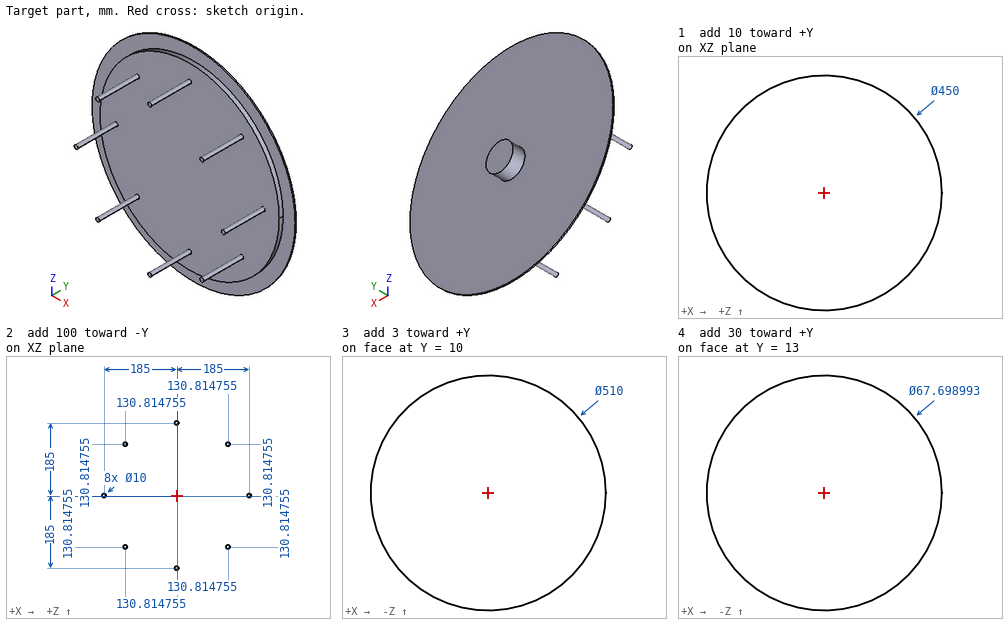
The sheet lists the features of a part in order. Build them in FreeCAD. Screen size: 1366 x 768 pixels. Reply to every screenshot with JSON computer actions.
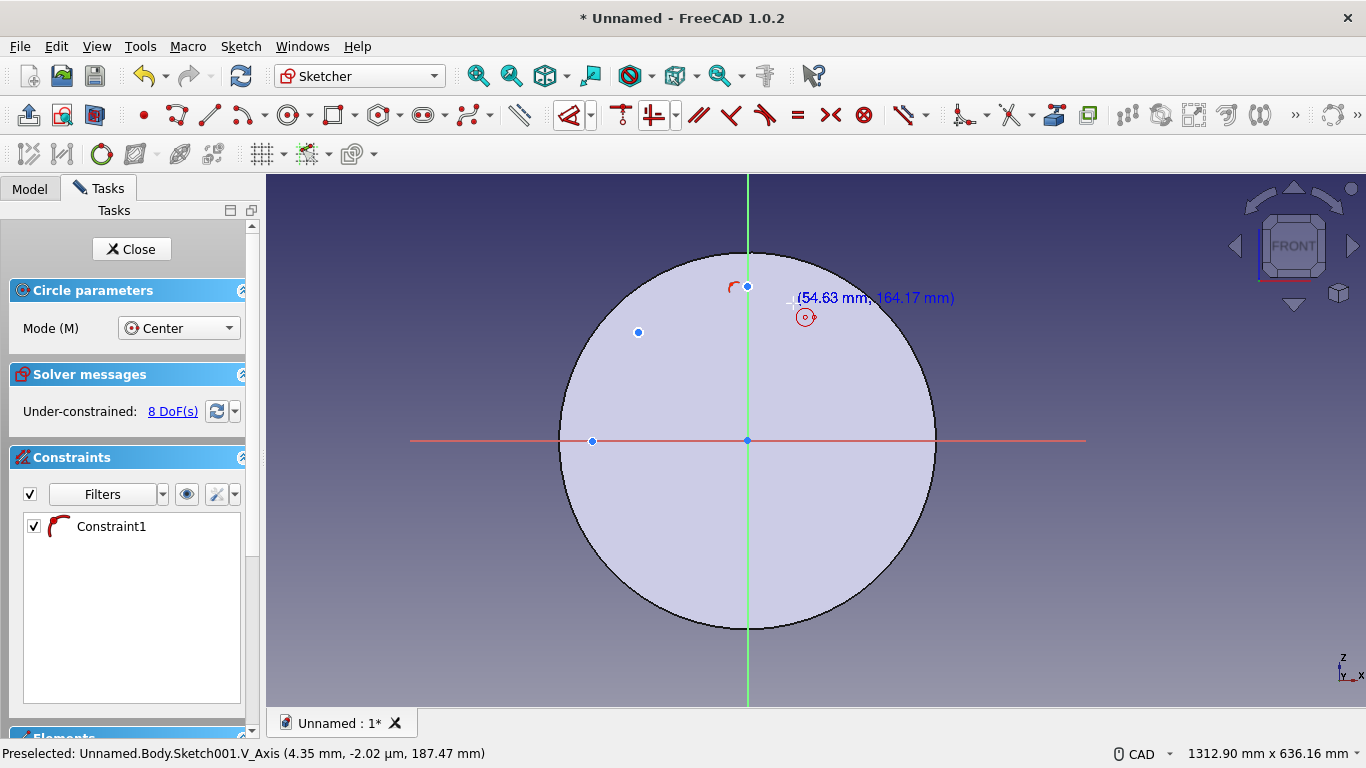
{"action": "left_click", "coordinate": [857, 331]}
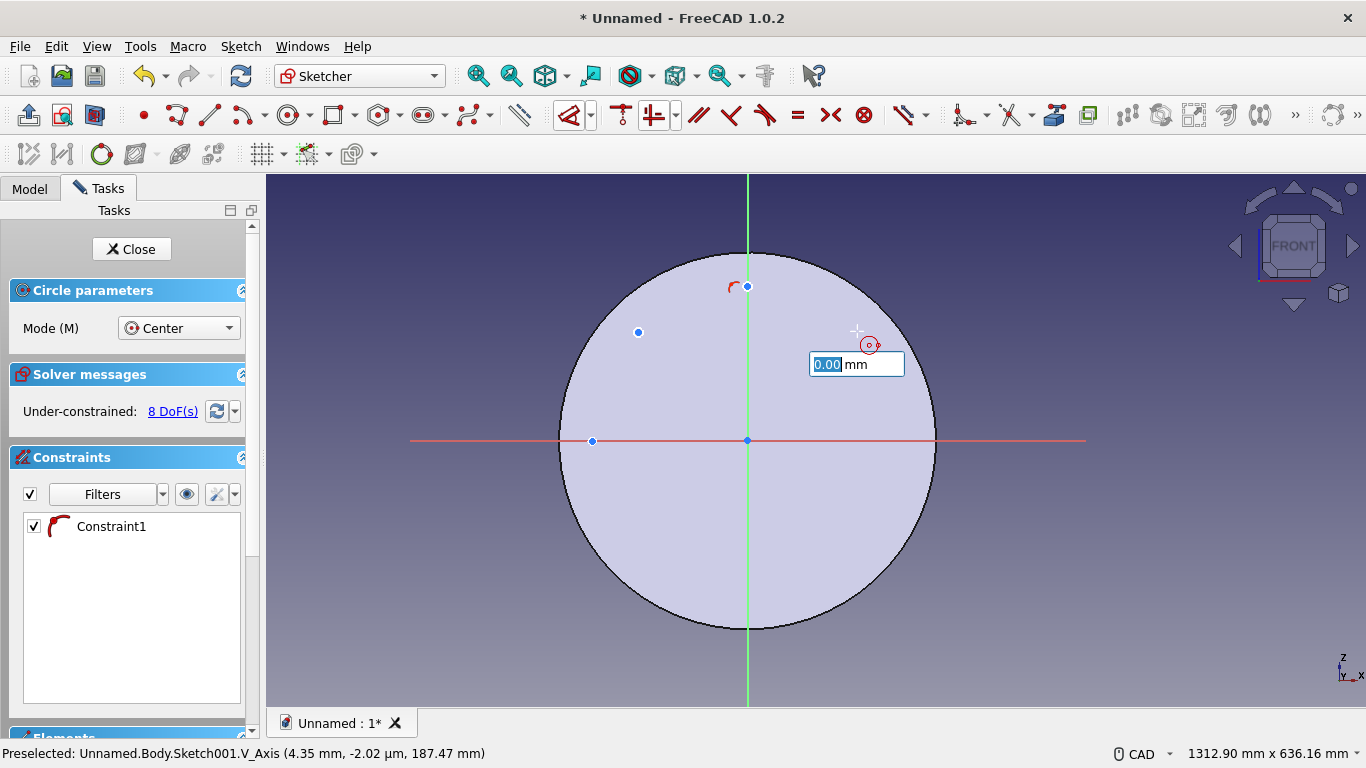
{"action": "scroll", "coordinate": [860, 328], "scroll_direction": "up", "scroll_amount": 7}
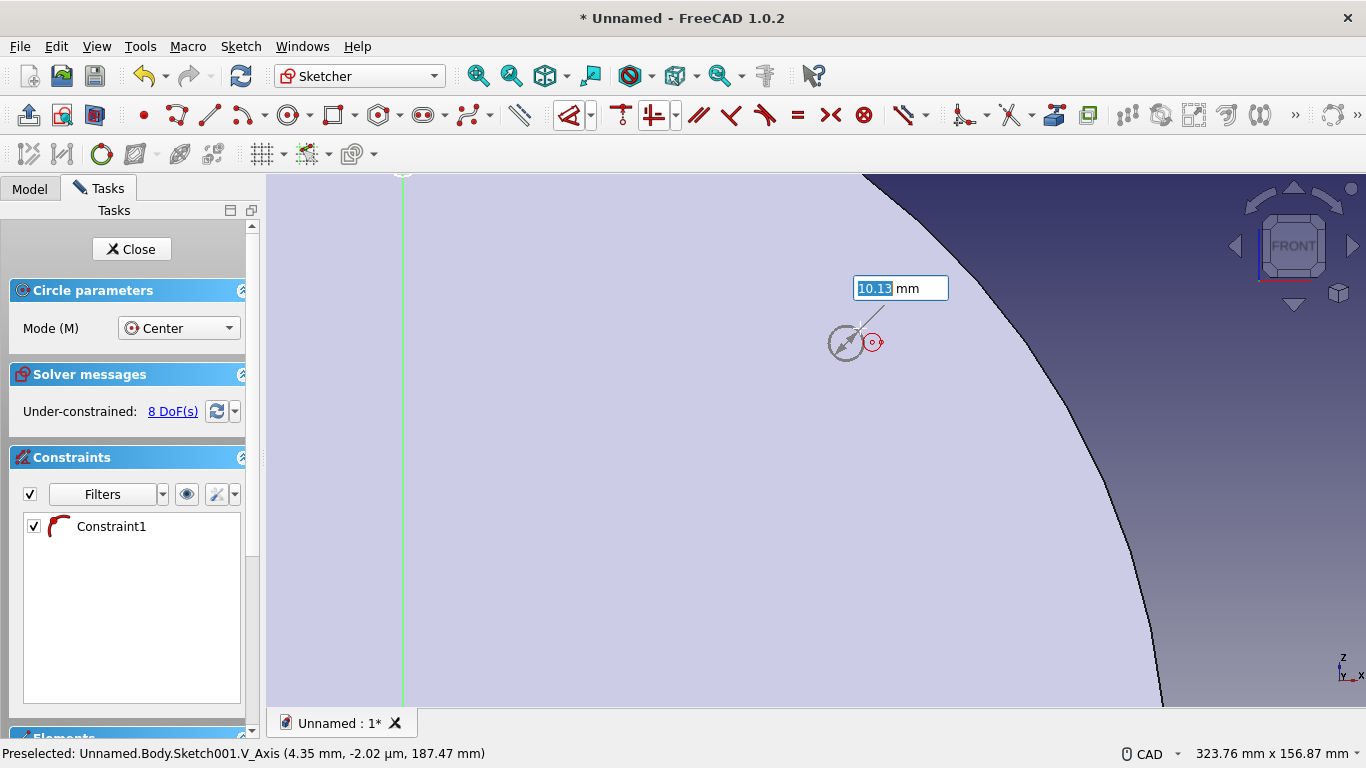
{"action": "left_click", "coordinate": [859, 329]}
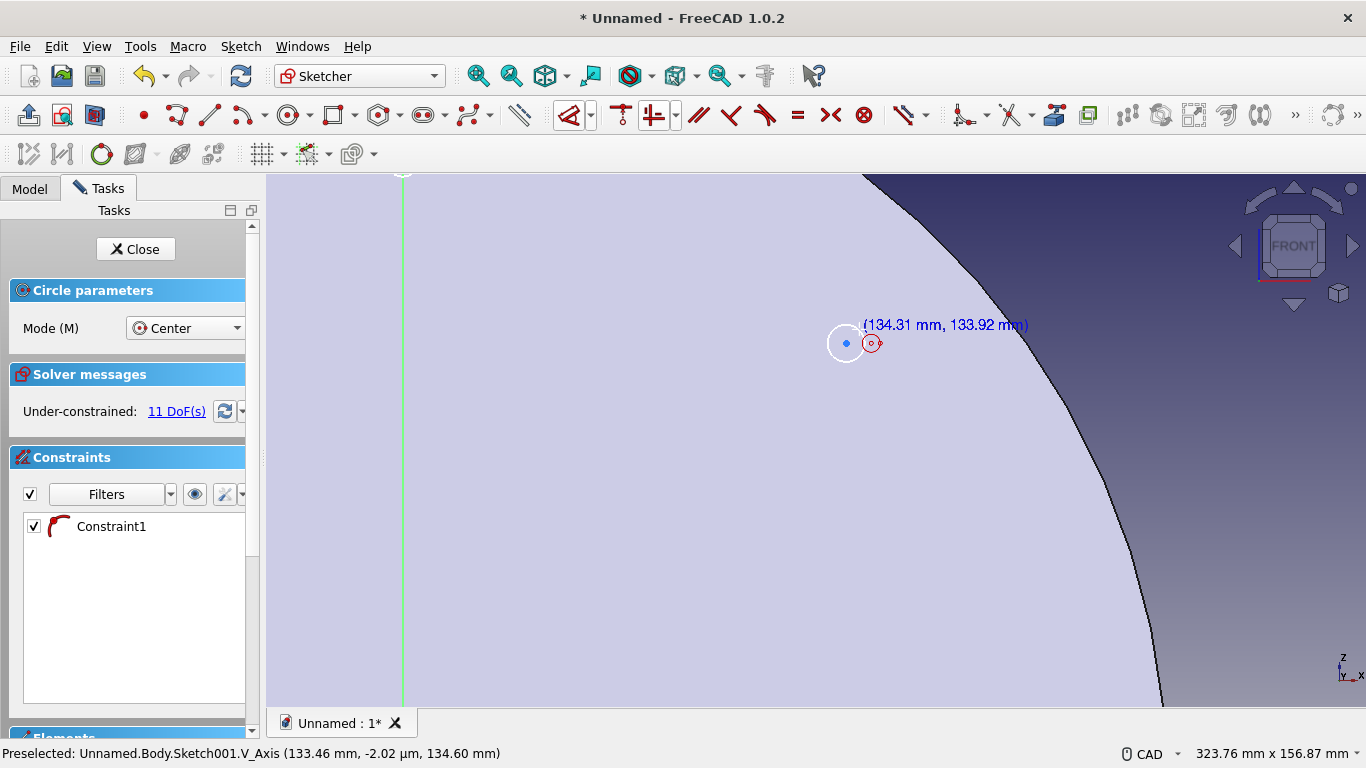
{"action": "scroll", "coordinate": [860, 328], "scroll_direction": "down", "scroll_amount": 7}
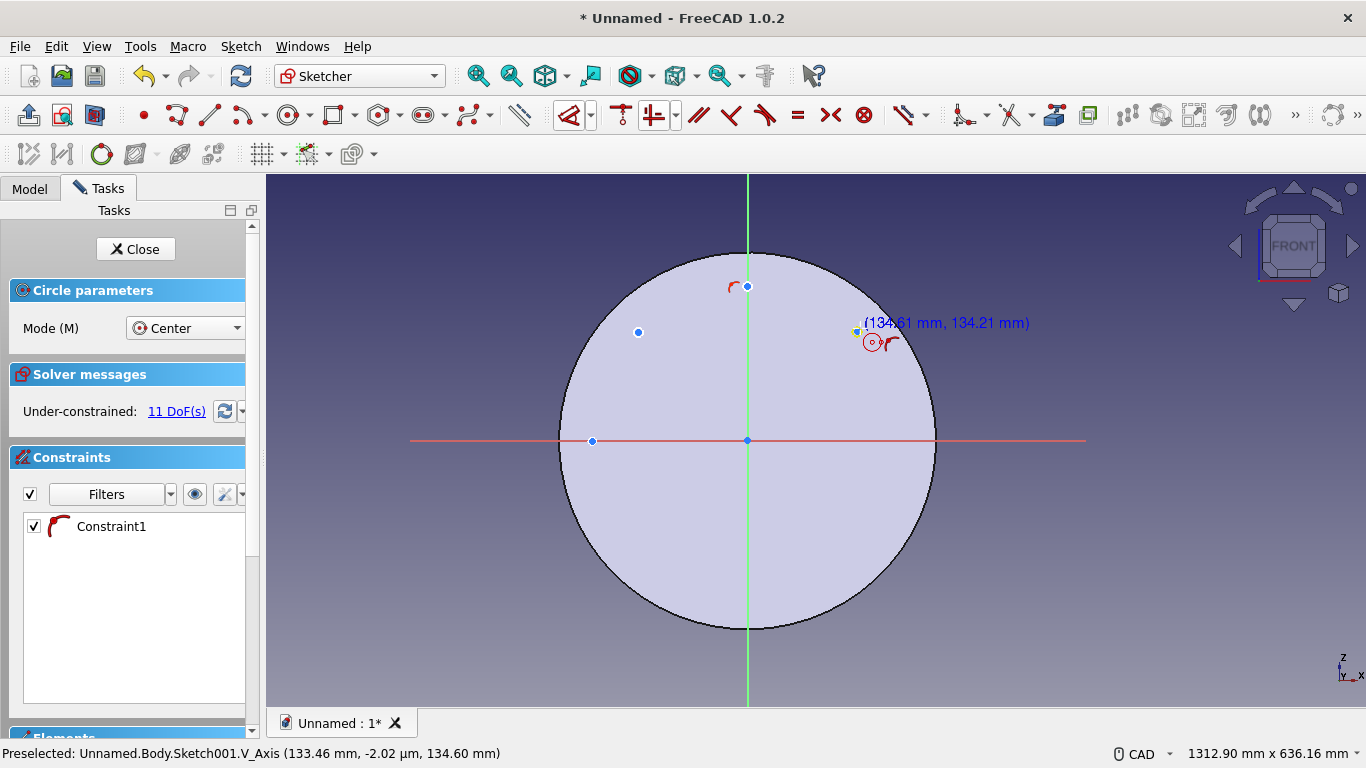
{"action": "scroll", "coordinate": [903, 441], "scroll_direction": "up", "scroll_amount": 9}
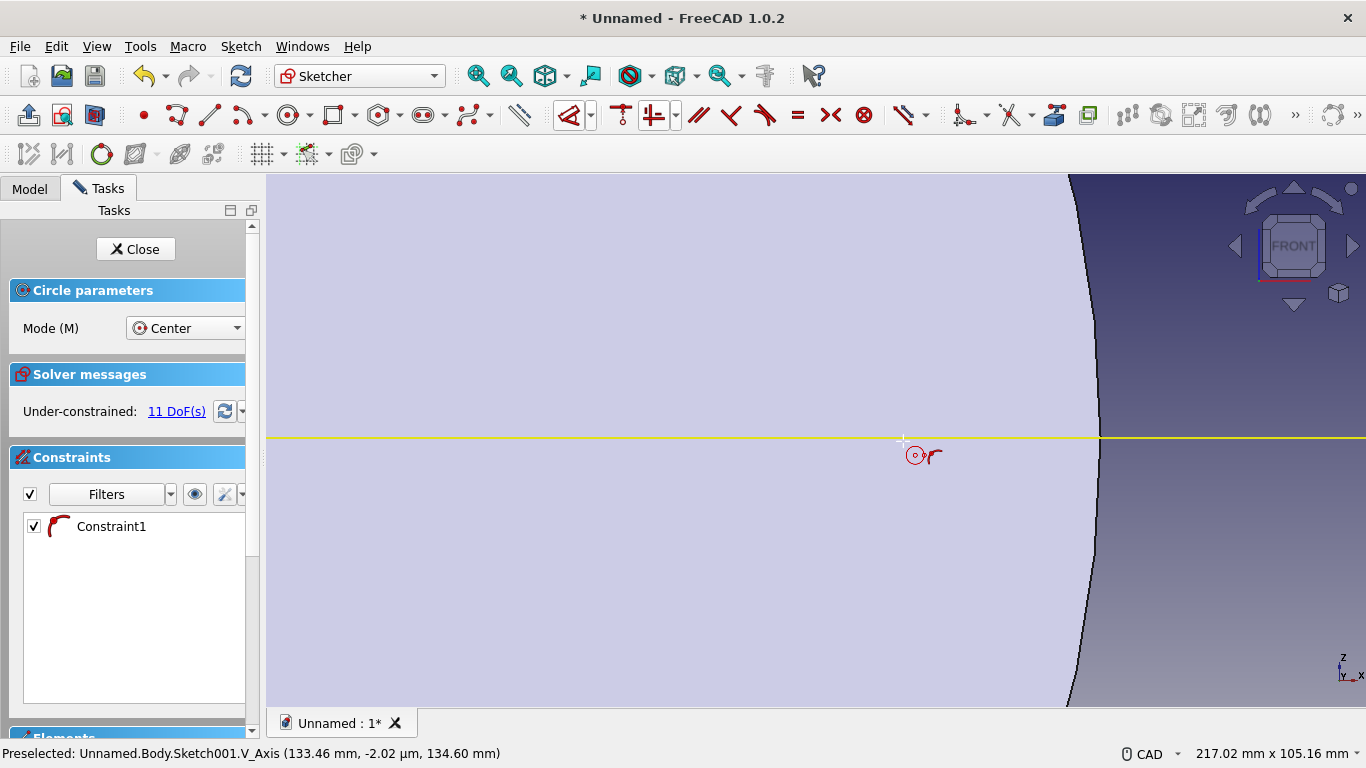
{"action": "scroll", "coordinate": [903, 441], "scroll_direction": "down", "scroll_amount": 9}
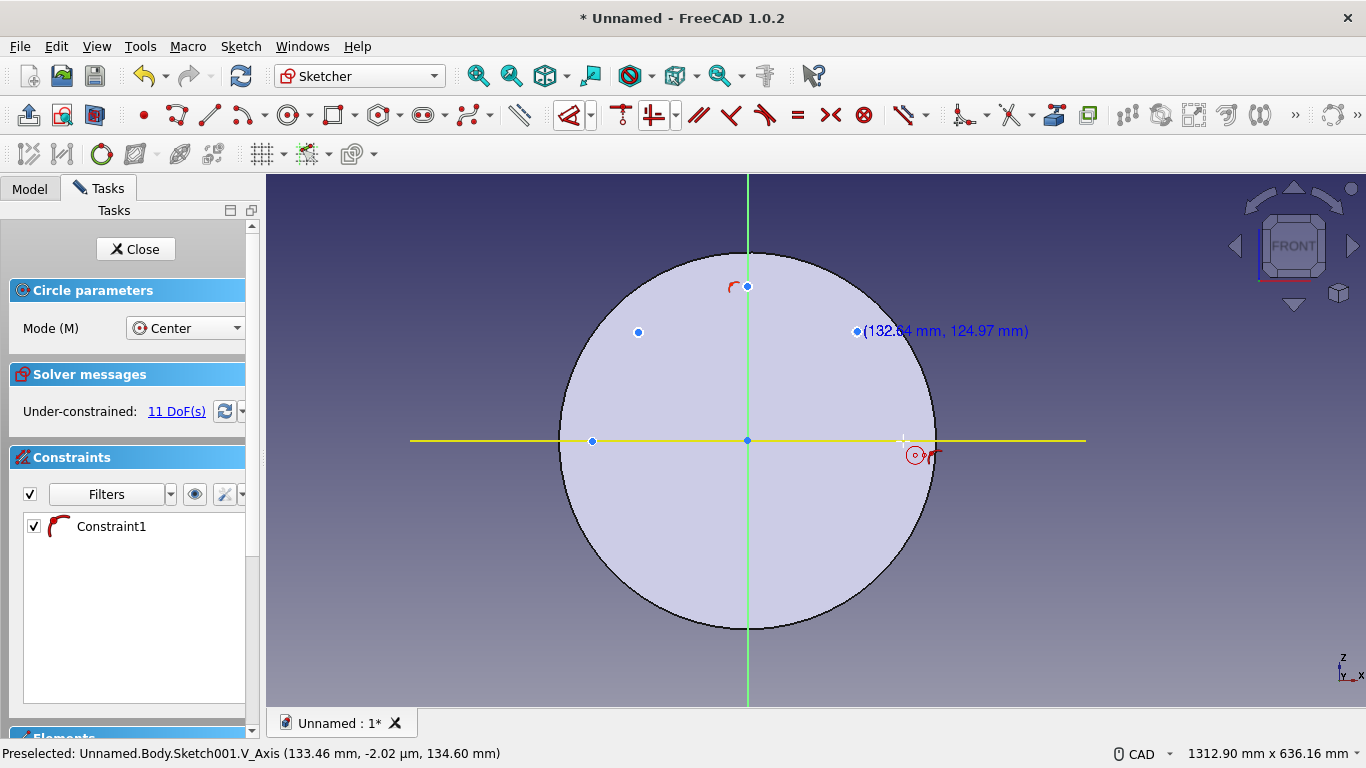
{"action": "left_click", "coordinate": [903, 441]}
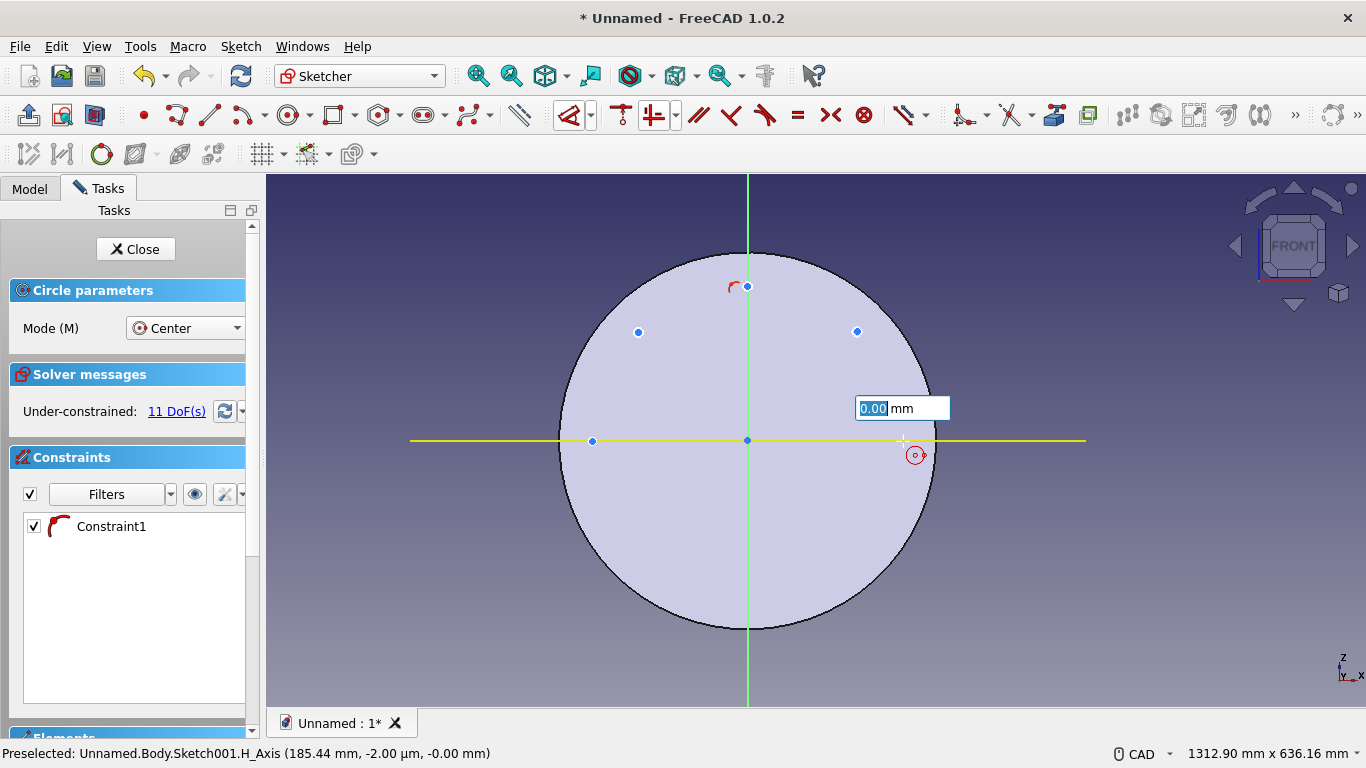
{"action": "scroll", "coordinate": [901, 445], "scroll_direction": "up", "scroll_amount": 7}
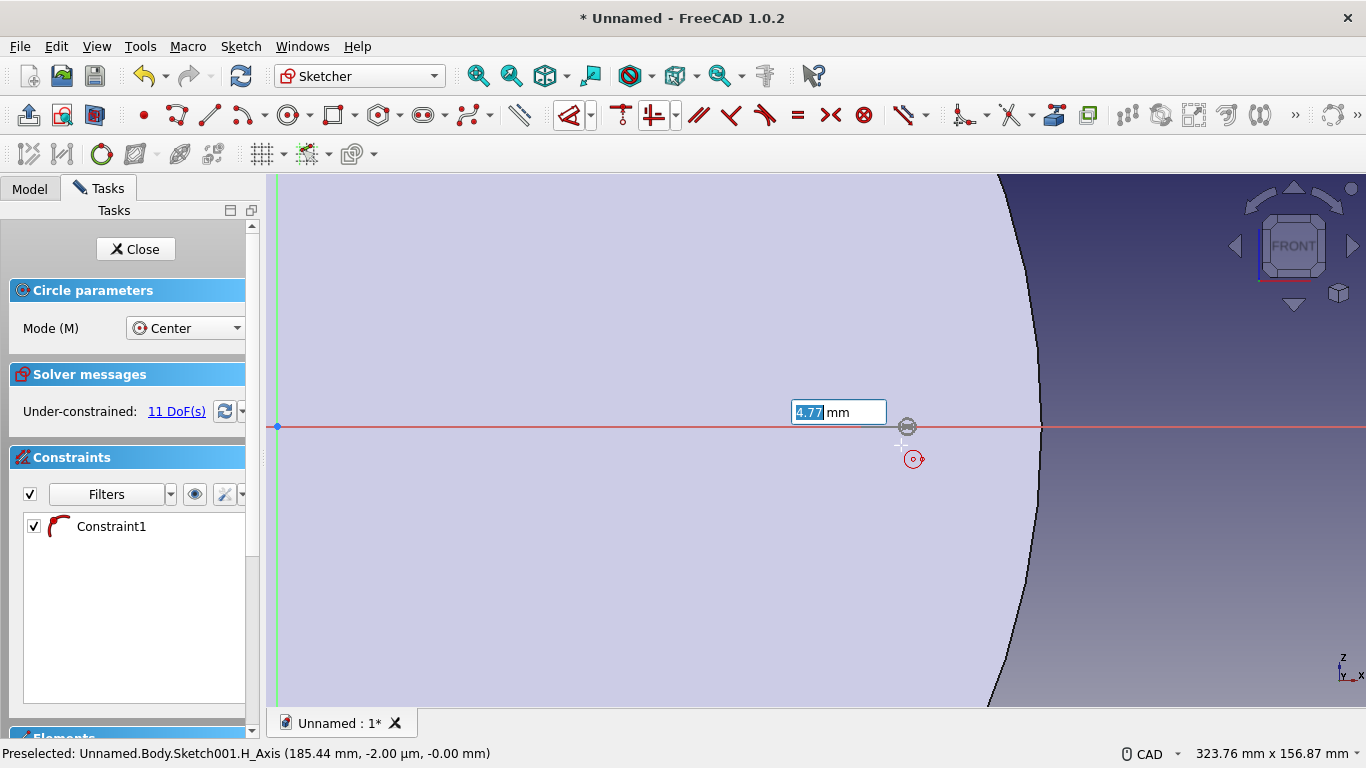
{"action": "left_click", "coordinate": [900, 443]}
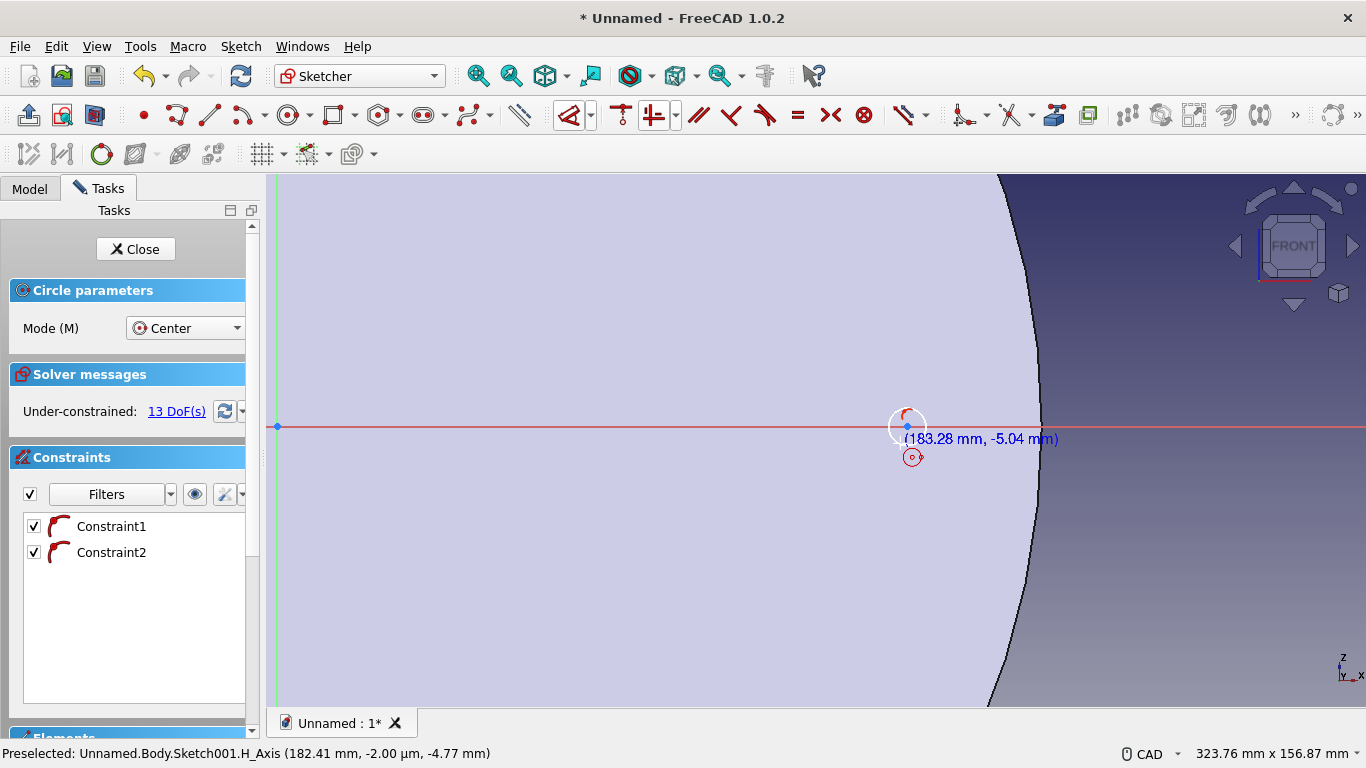
{"action": "scroll", "coordinate": [901, 445], "scroll_direction": "down", "scroll_amount": 7}